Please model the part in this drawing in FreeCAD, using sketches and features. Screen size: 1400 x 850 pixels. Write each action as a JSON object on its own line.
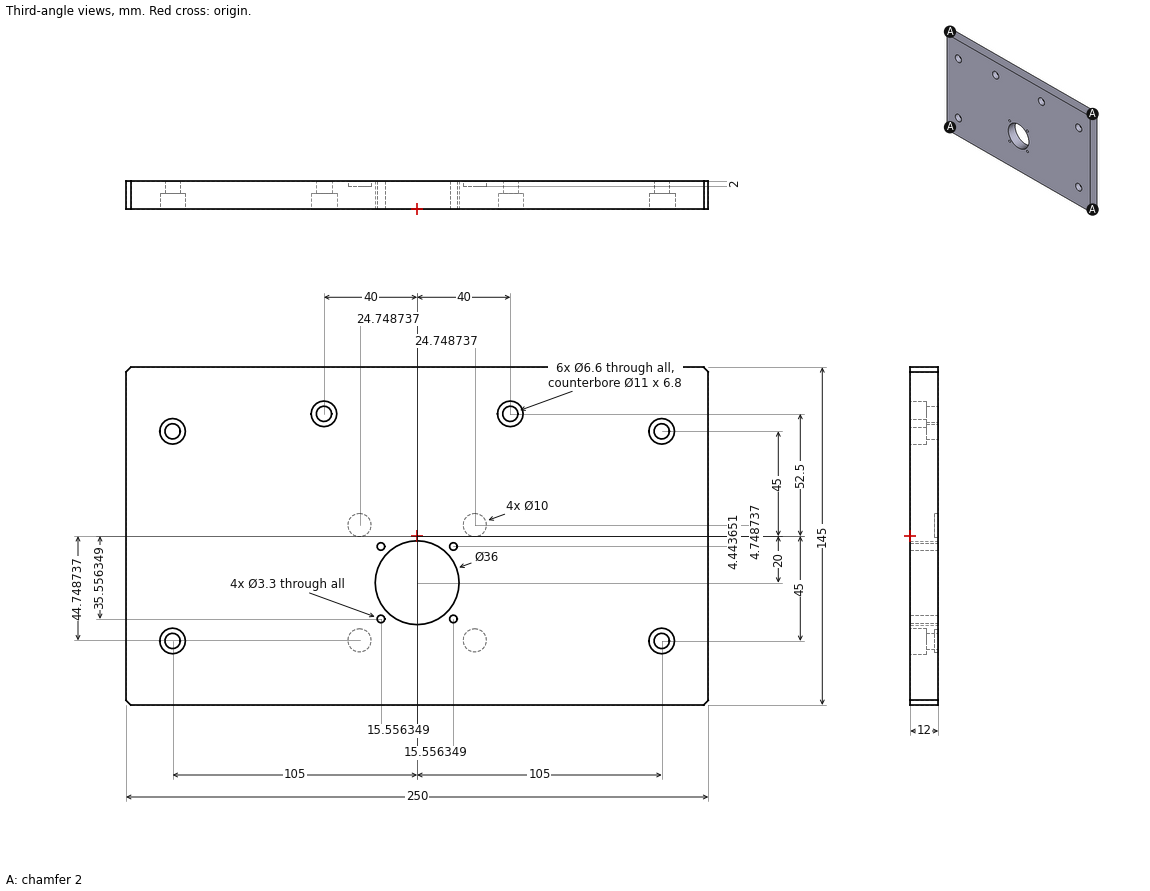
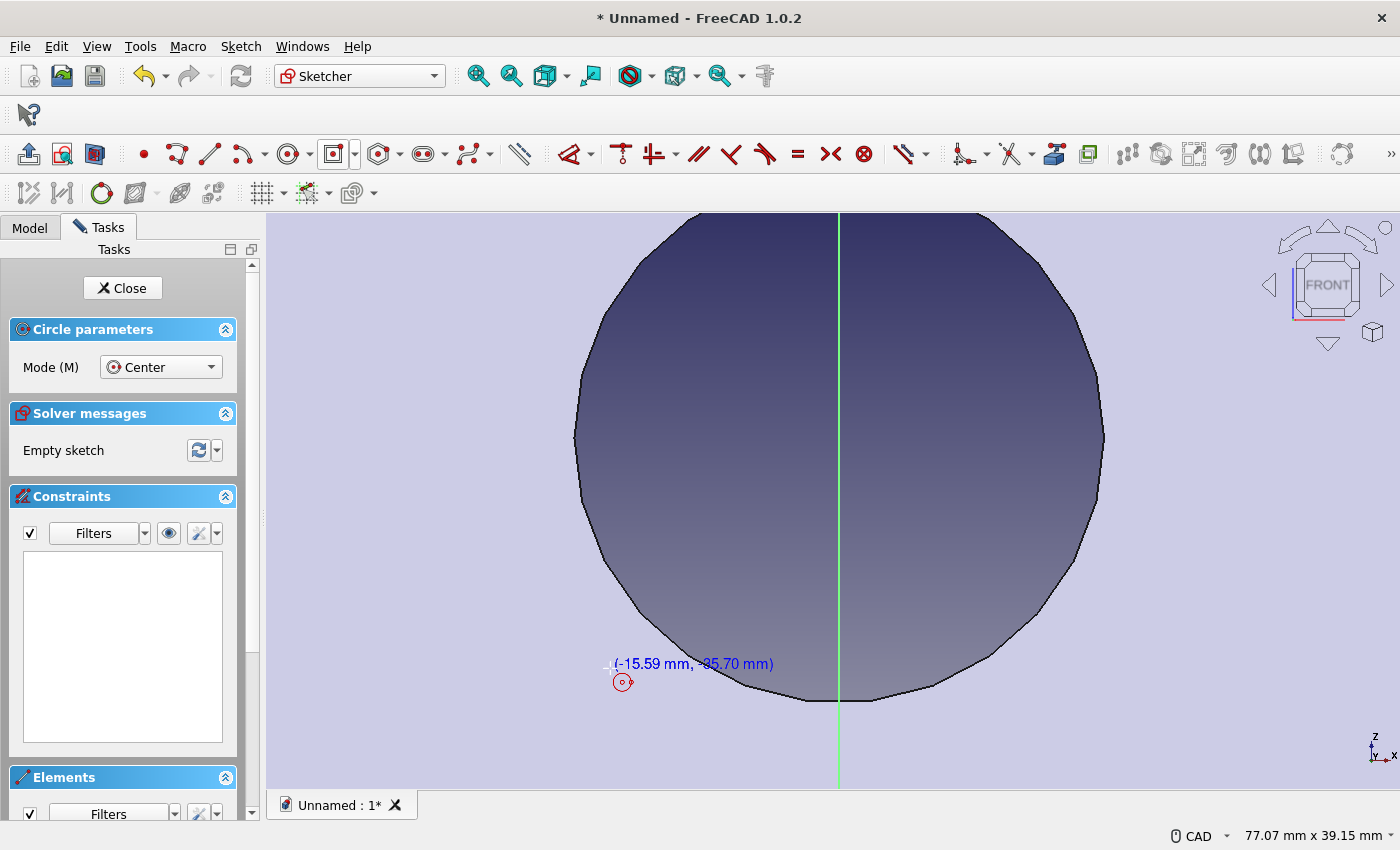
{"action": "left_click", "coordinate": [610, 667]}
{"action": "mouse_move", "coordinate": [628, 650]}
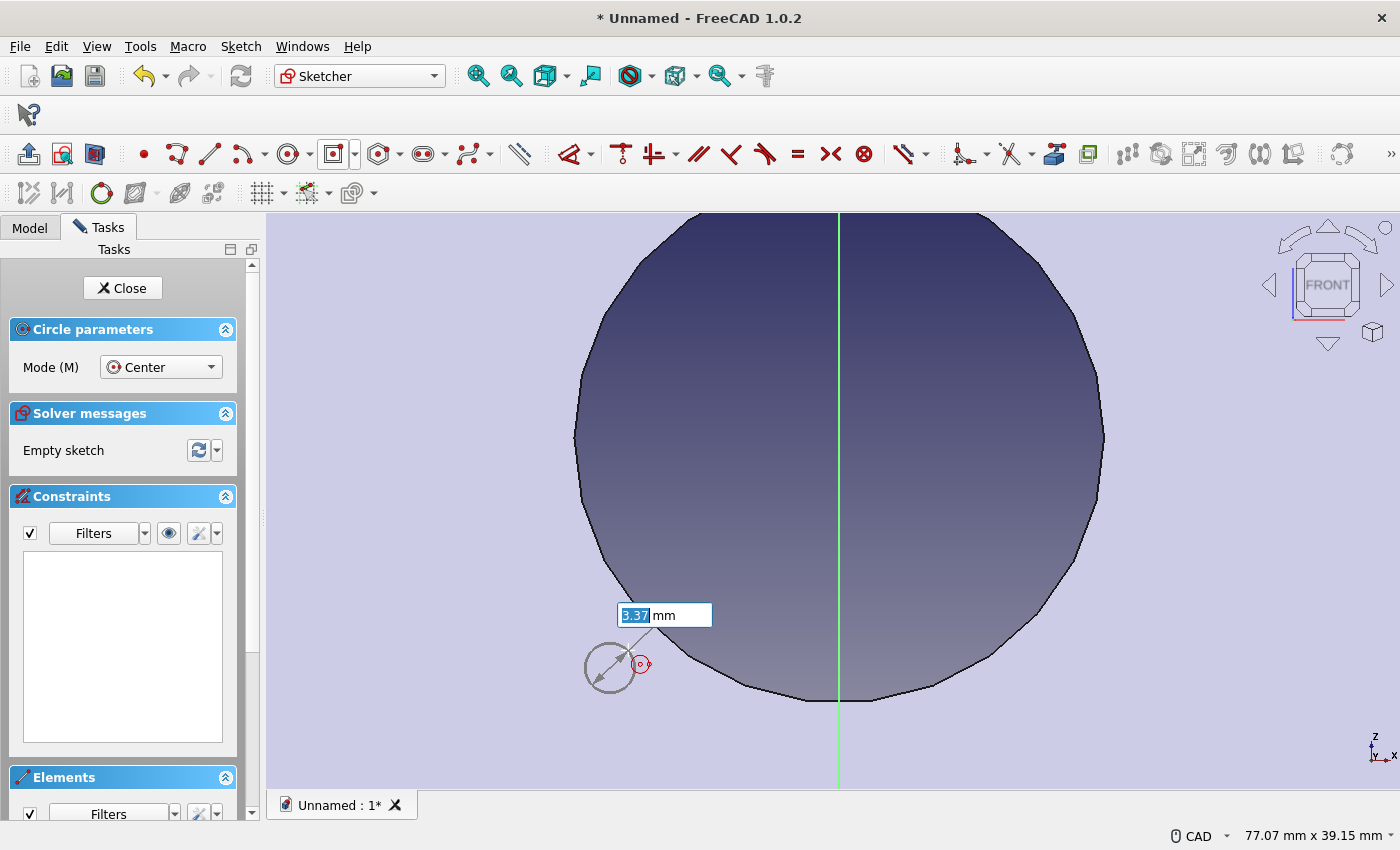
{"action": "type", "text": "3.3"}
{"action": "key", "text": "Return"}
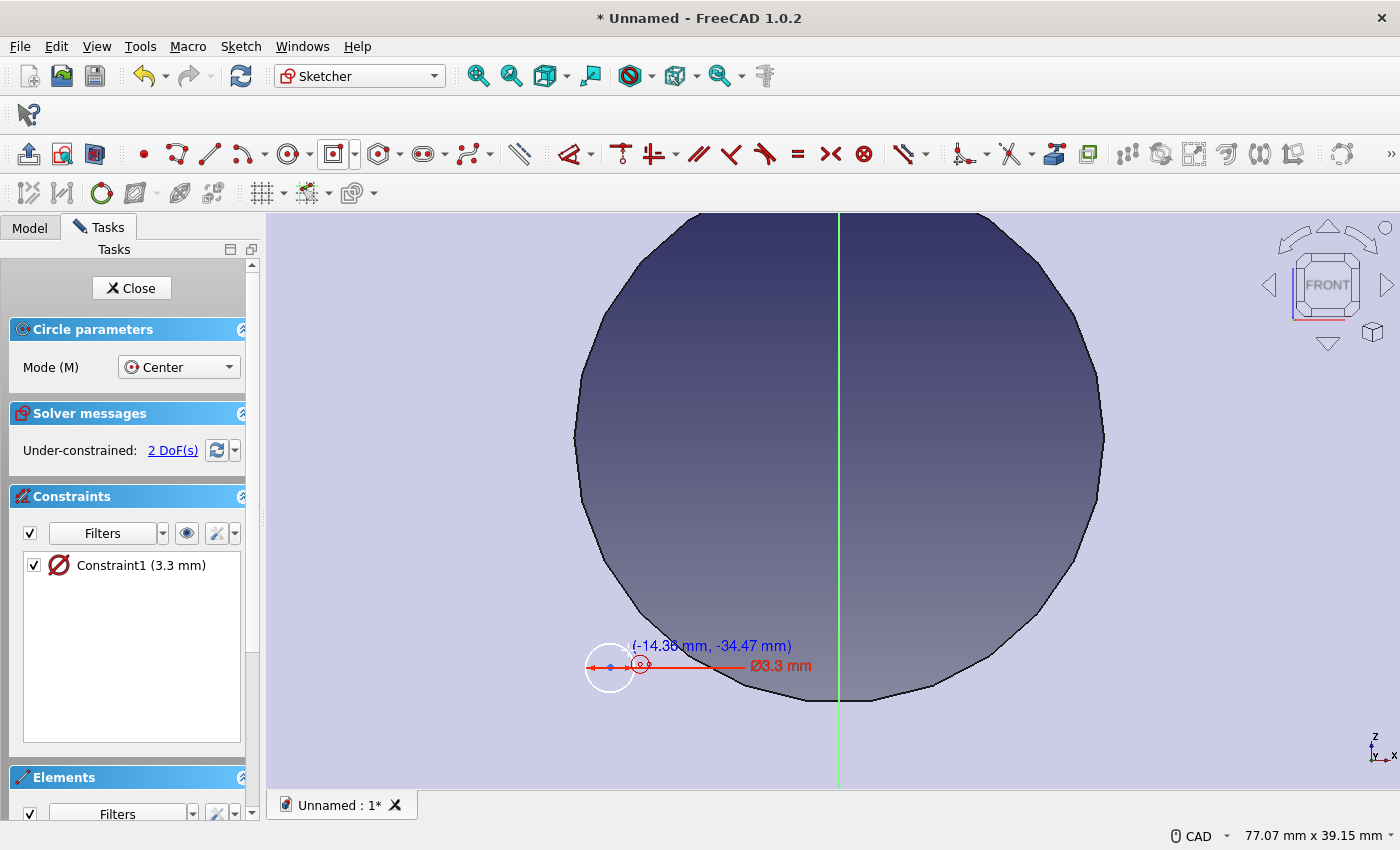
{"action": "left_click", "coordinate": [1068, 667]}
{"action": "mouse_move", "coordinate": [1085, 650]}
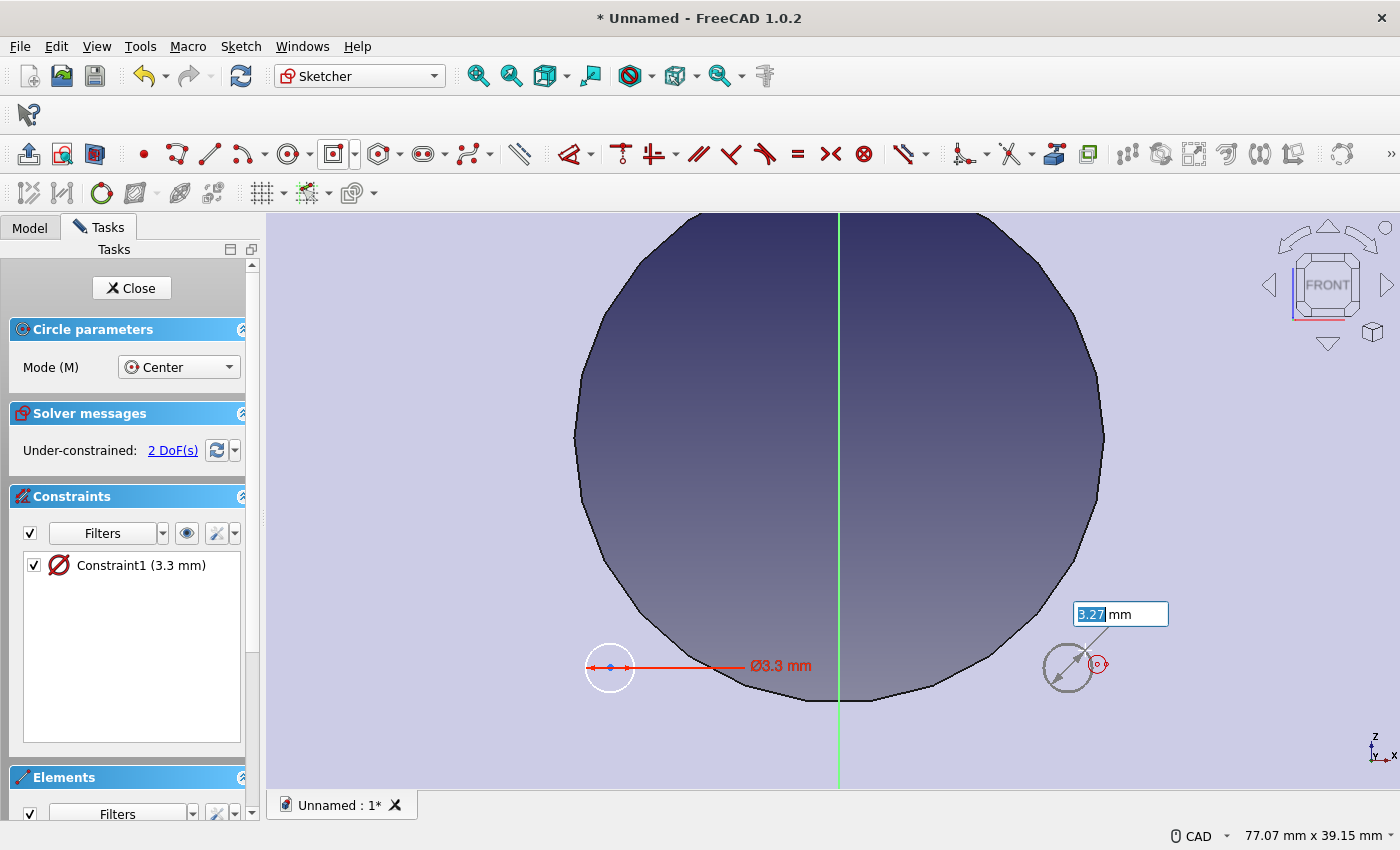
{"action": "type", "text": "3.3"}
{"action": "key", "text": "Return"}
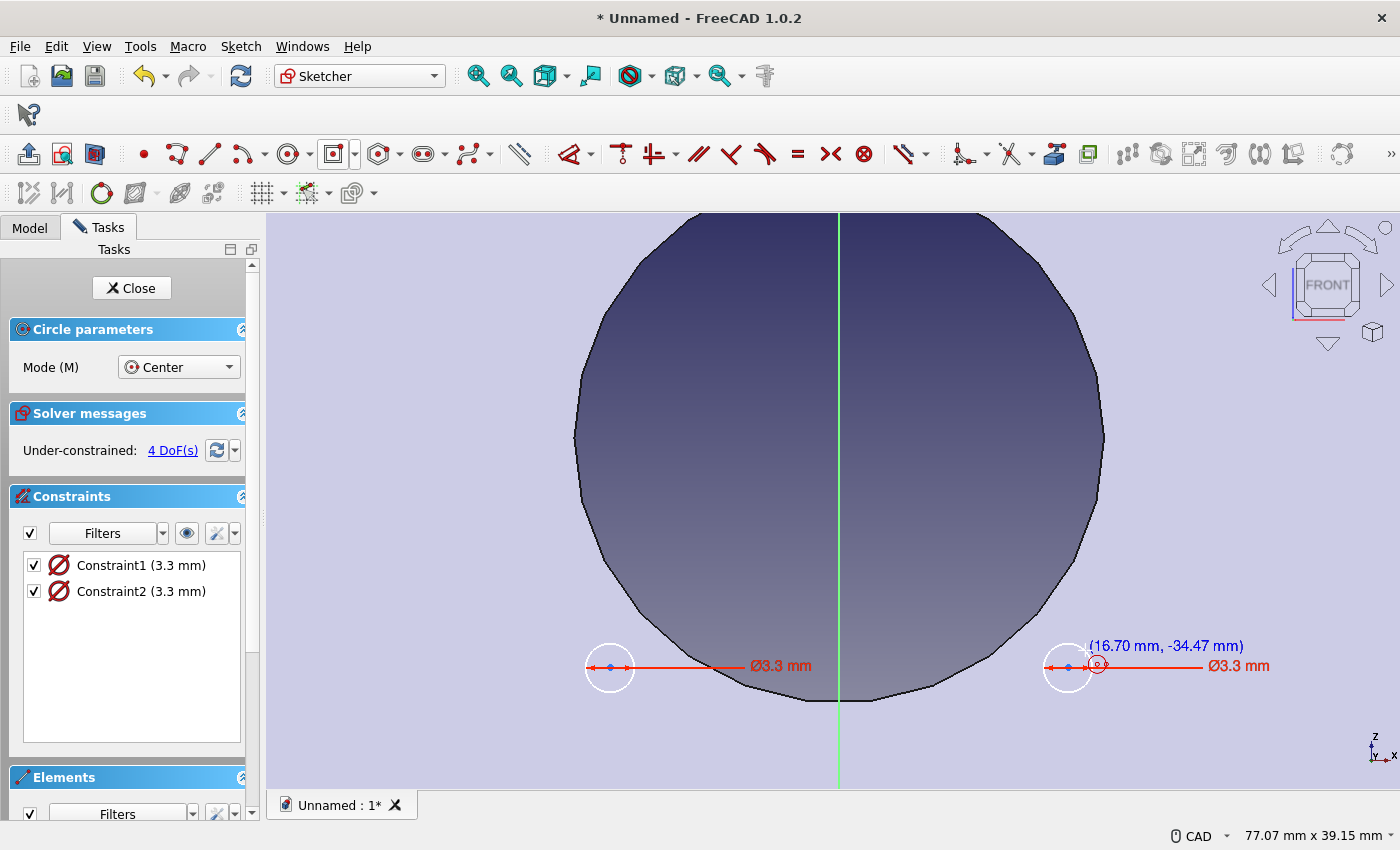
{"action": "scroll", "coordinate": [613, 671], "scroll_direction": "down", "scroll_amount": 2}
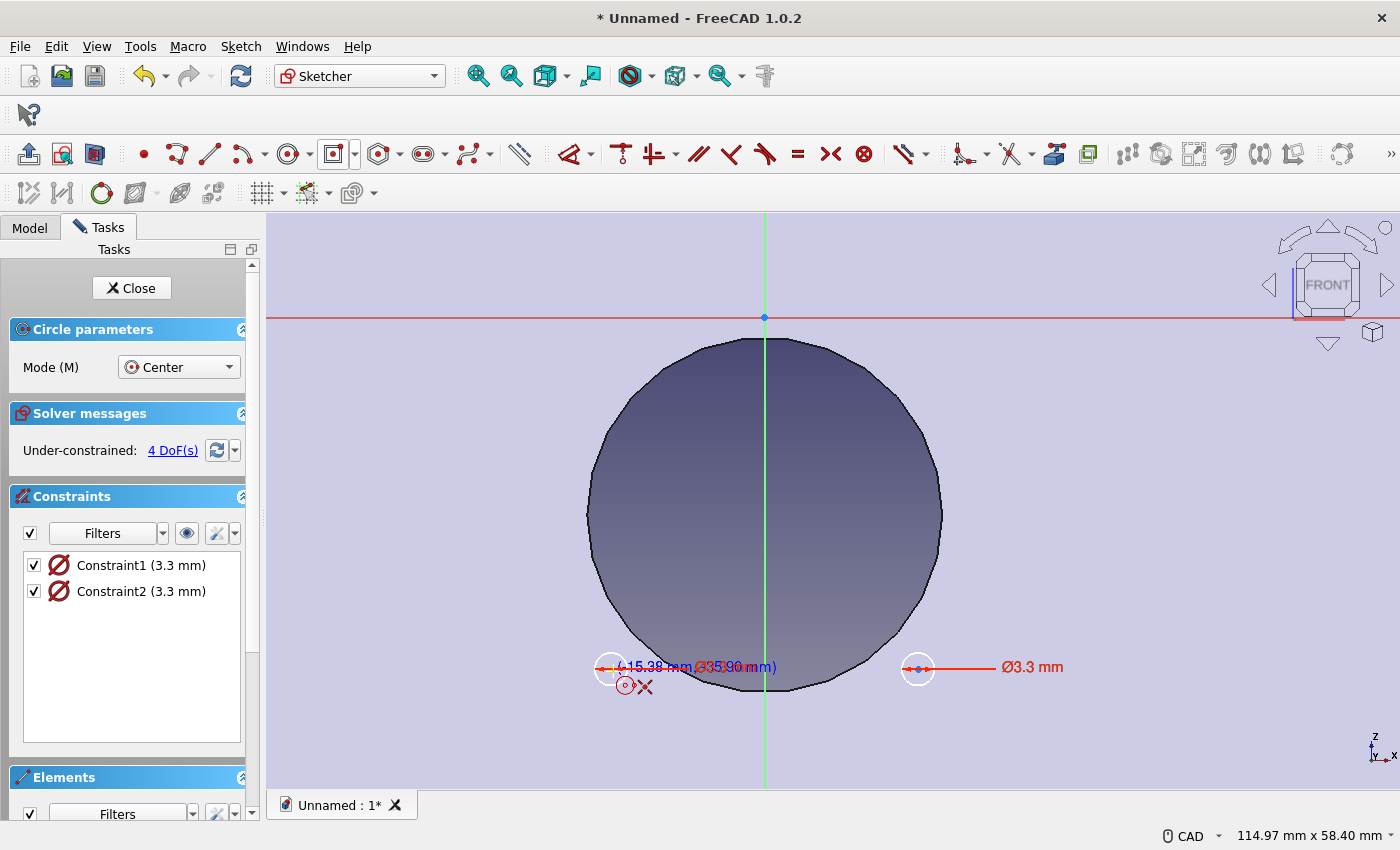
{"action": "scroll", "coordinate": [918, 362], "scroll_direction": "up", "scroll_amount": 2}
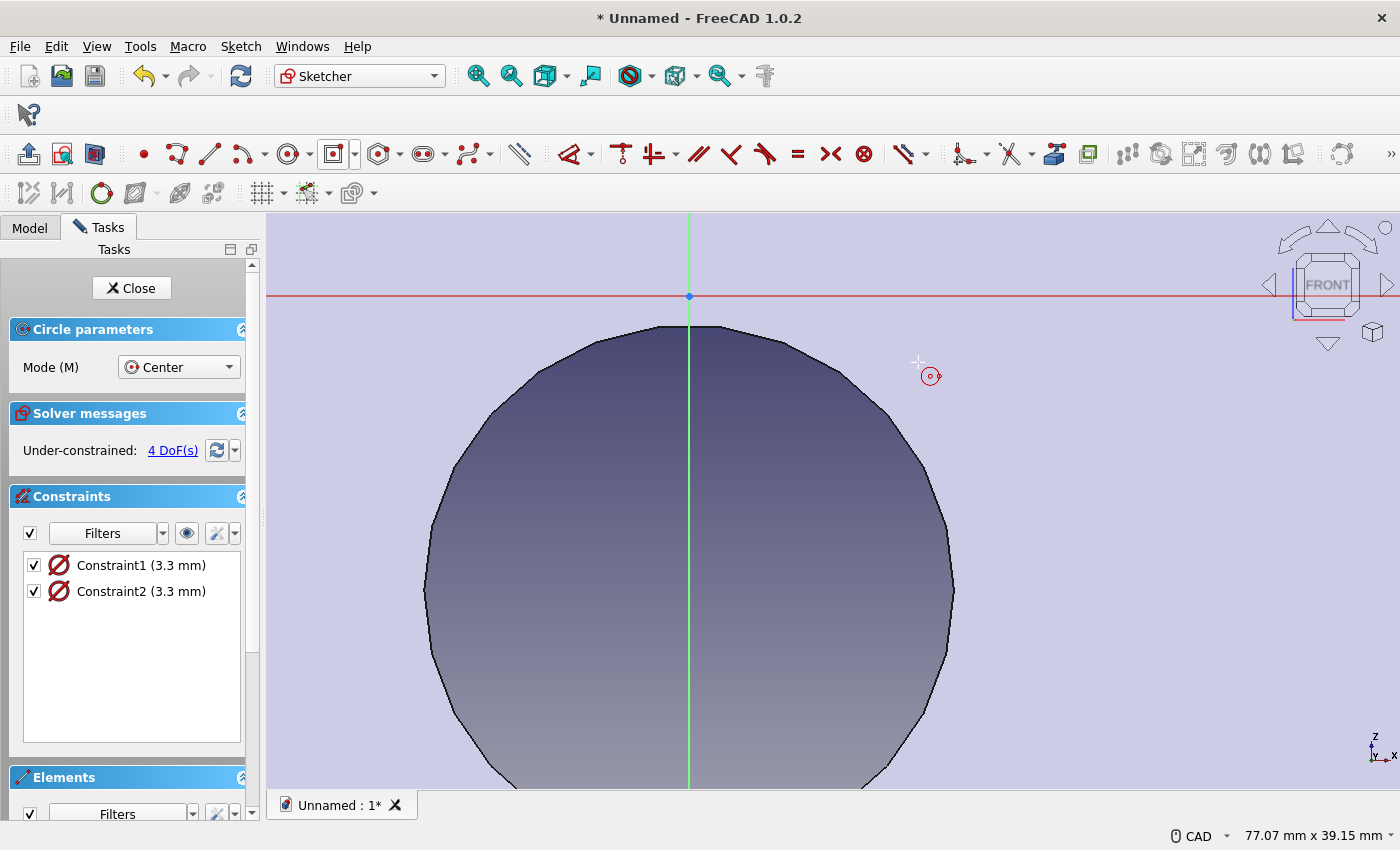
{"action": "left_click", "coordinate": [918, 361]}
{"action": "mouse_move", "coordinate": [935, 344]}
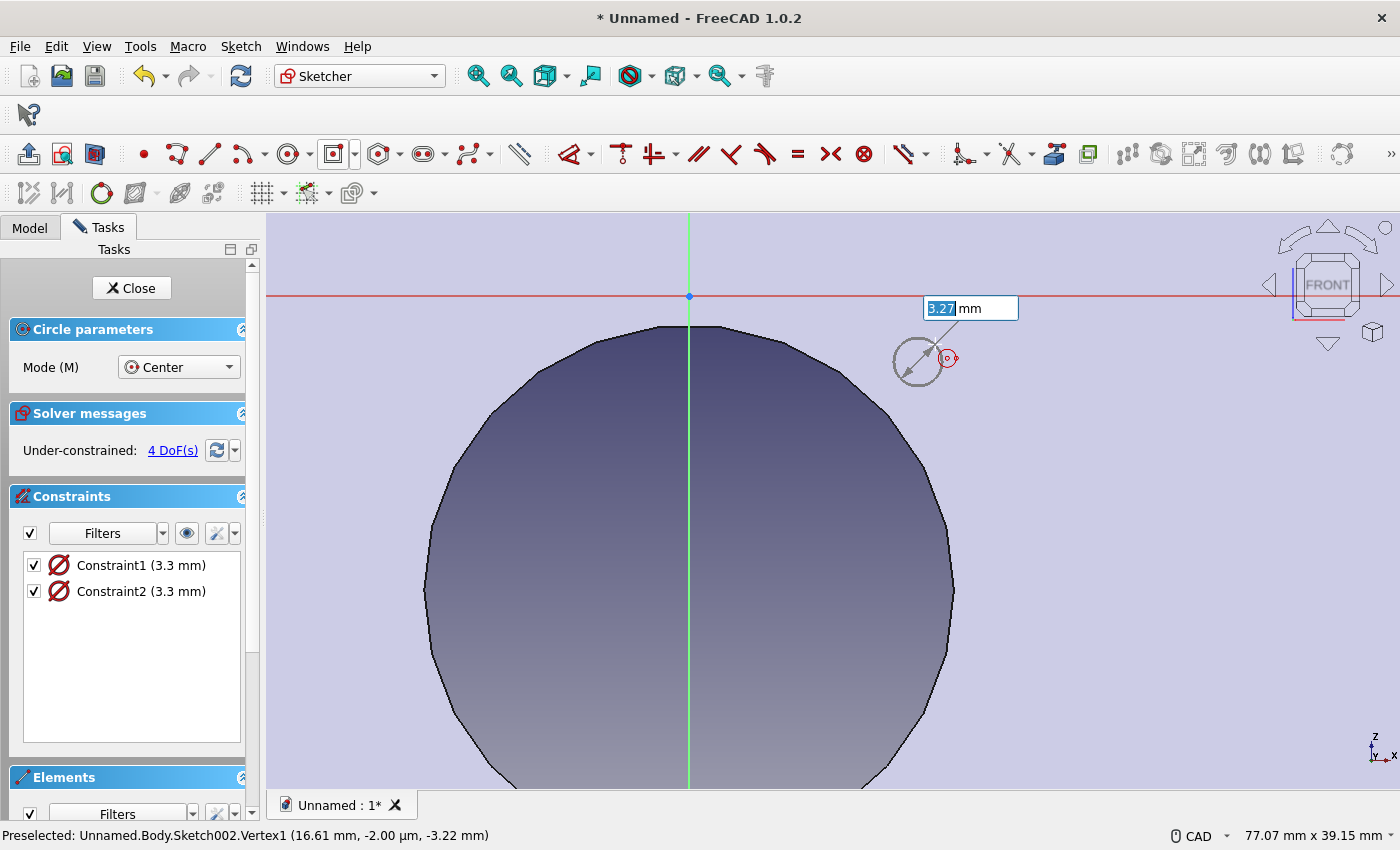
{"action": "type", "text": "3.3"}
{"action": "key", "text": "Return"}